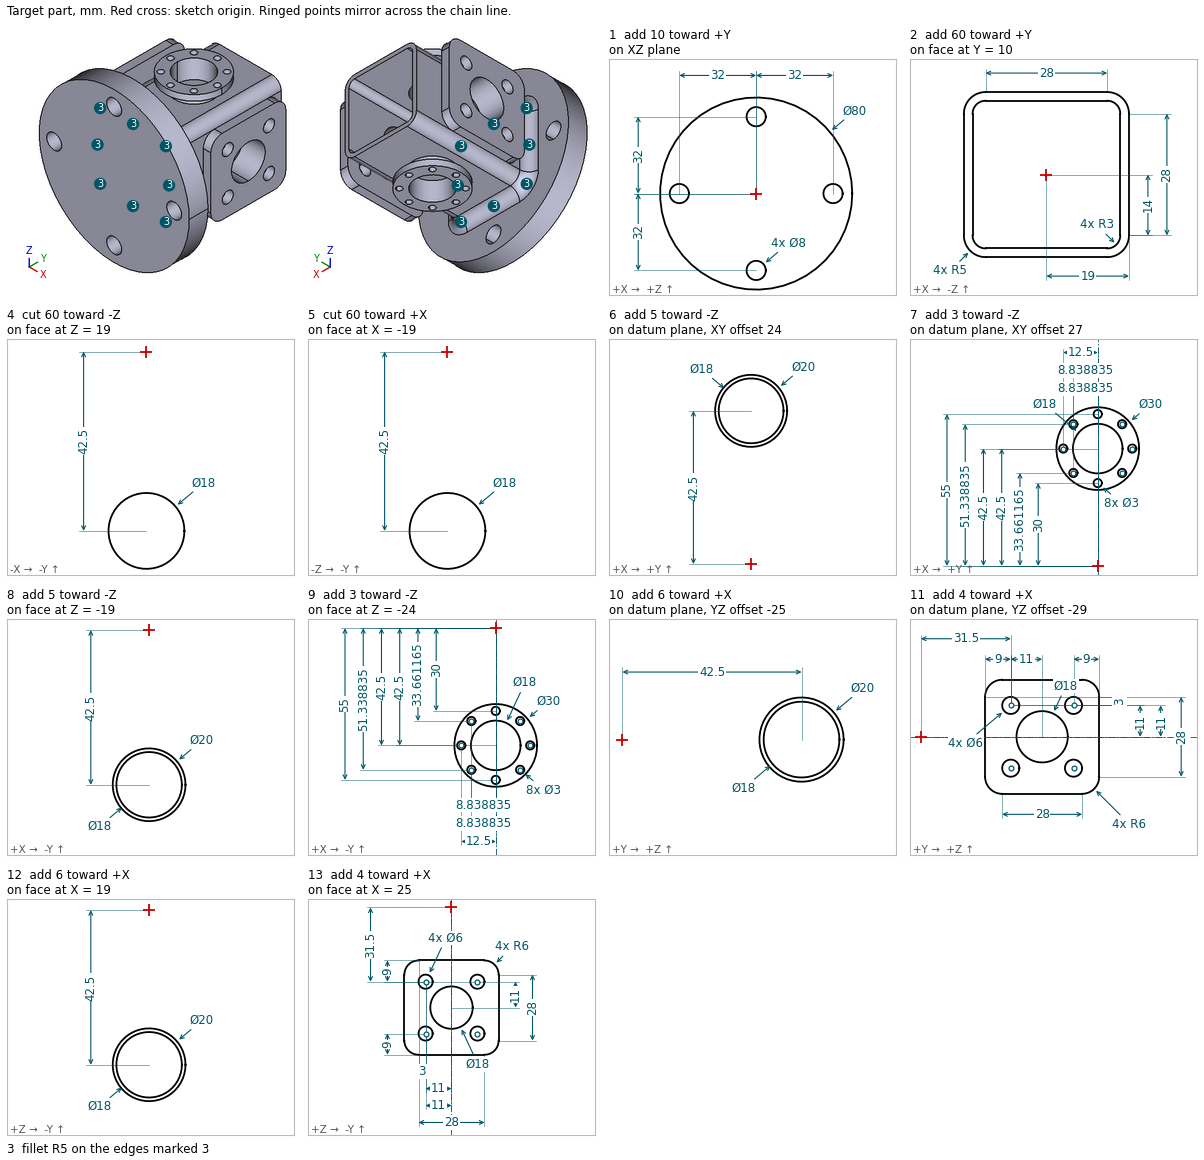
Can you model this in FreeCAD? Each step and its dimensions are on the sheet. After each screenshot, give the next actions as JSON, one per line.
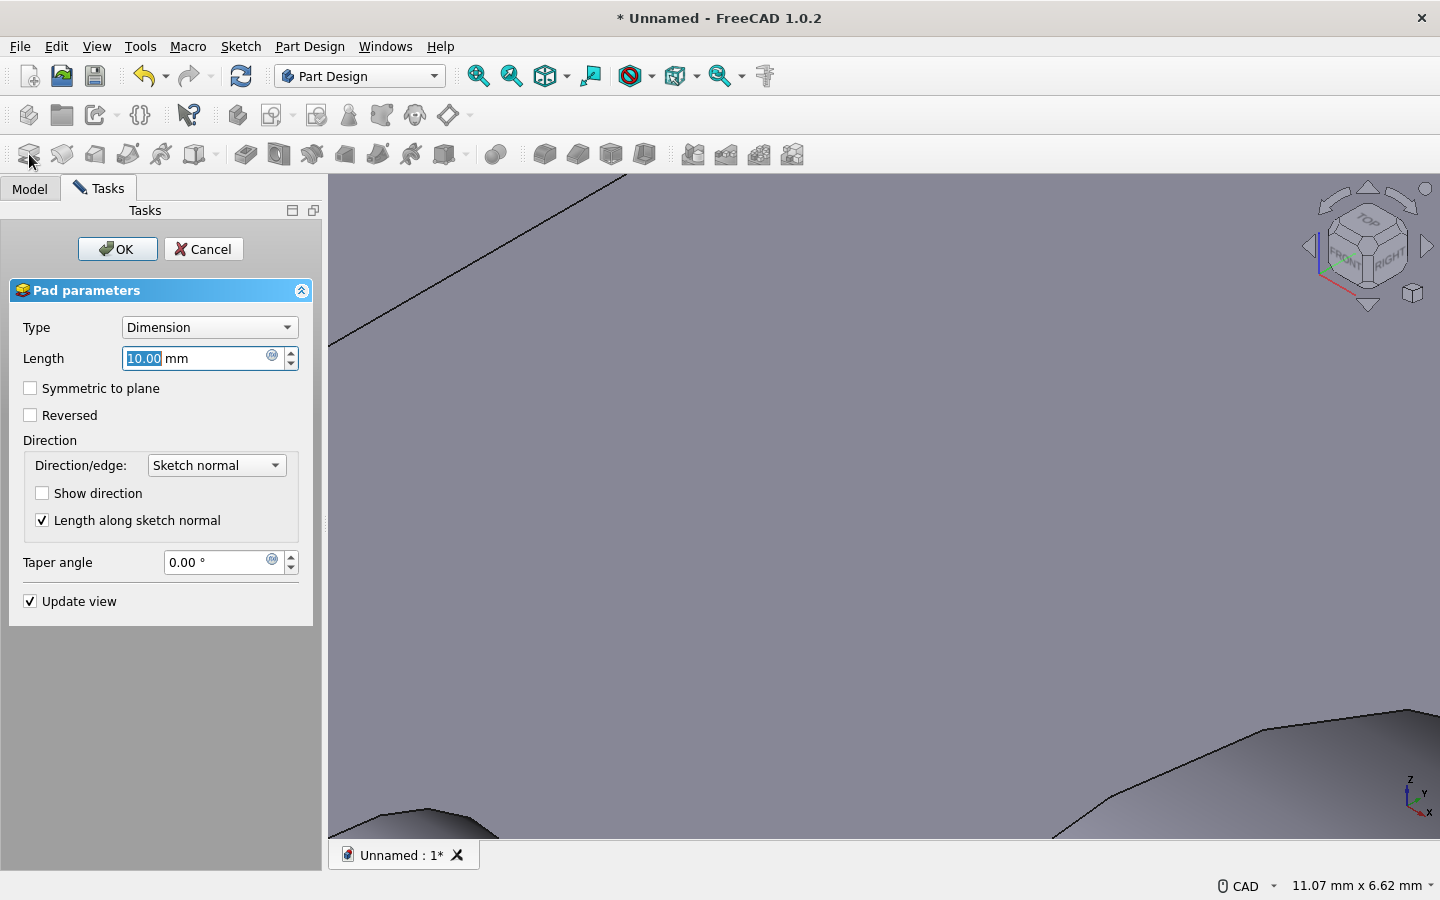
{"action": "type", "text": "4"}
{"action": "key", "text": "Tab"}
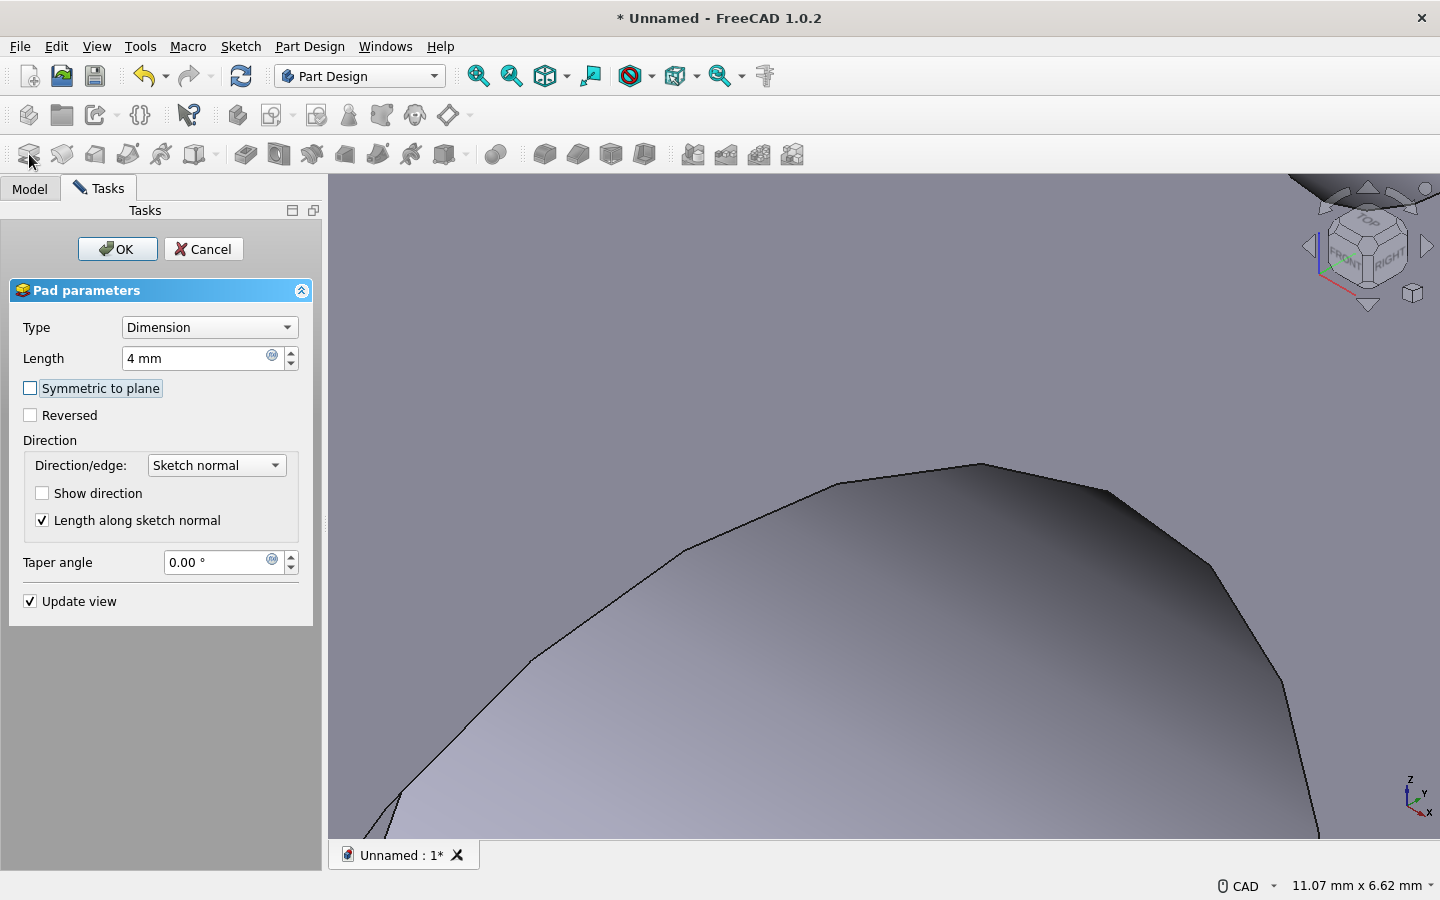
{"action": "left_click", "coordinate": [118, 249]}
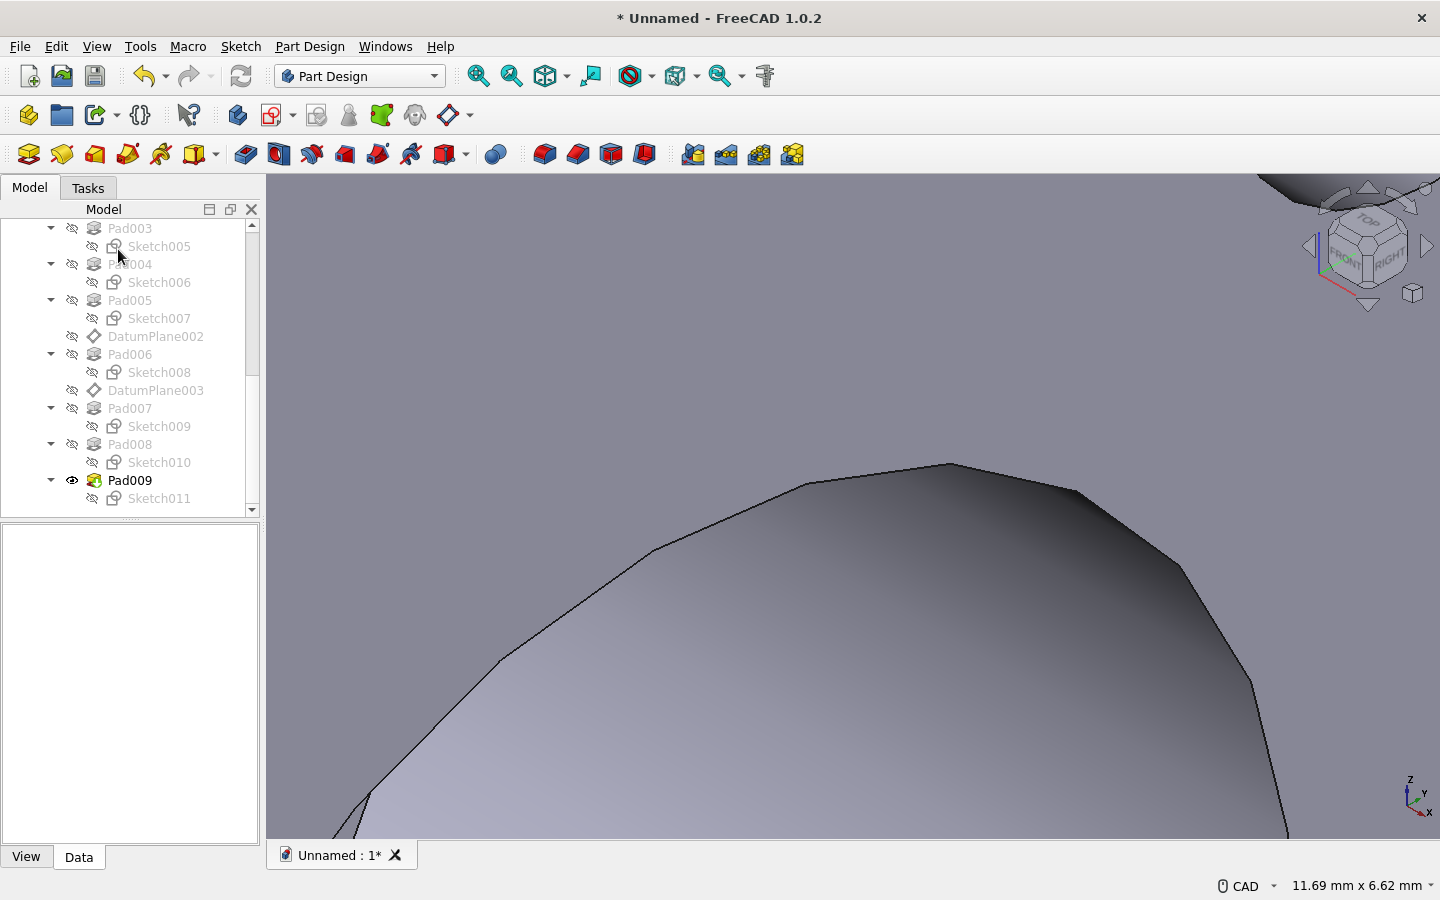
{"action": "key", "text": "v f"}